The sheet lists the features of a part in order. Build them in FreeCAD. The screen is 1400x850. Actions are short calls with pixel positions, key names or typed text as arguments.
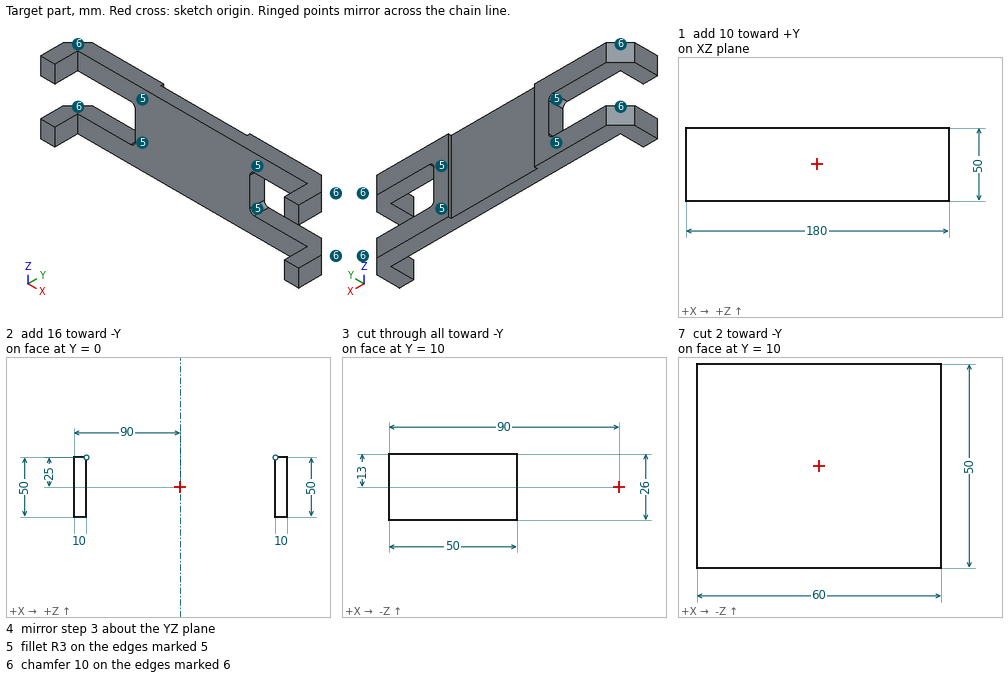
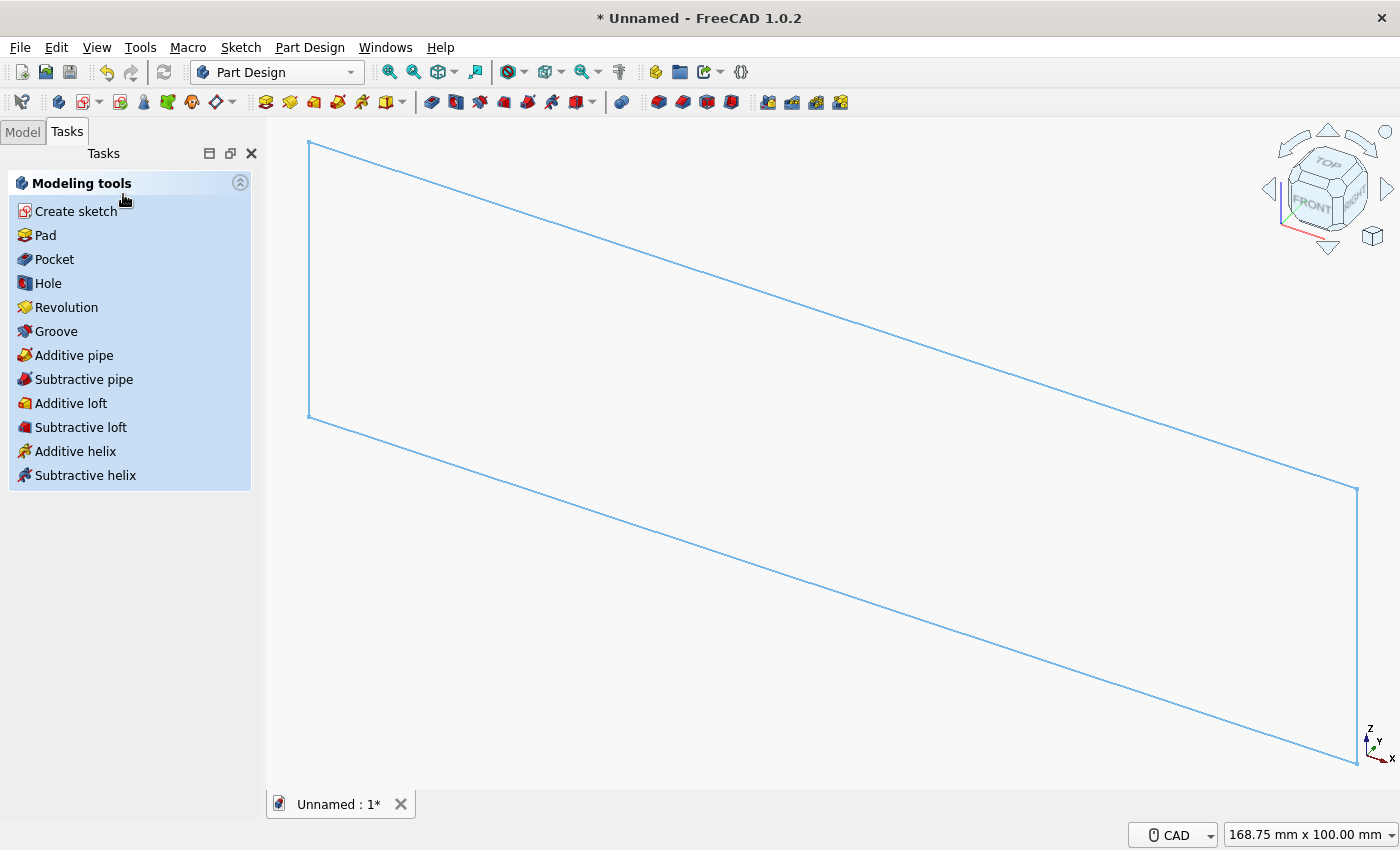
click(266, 102)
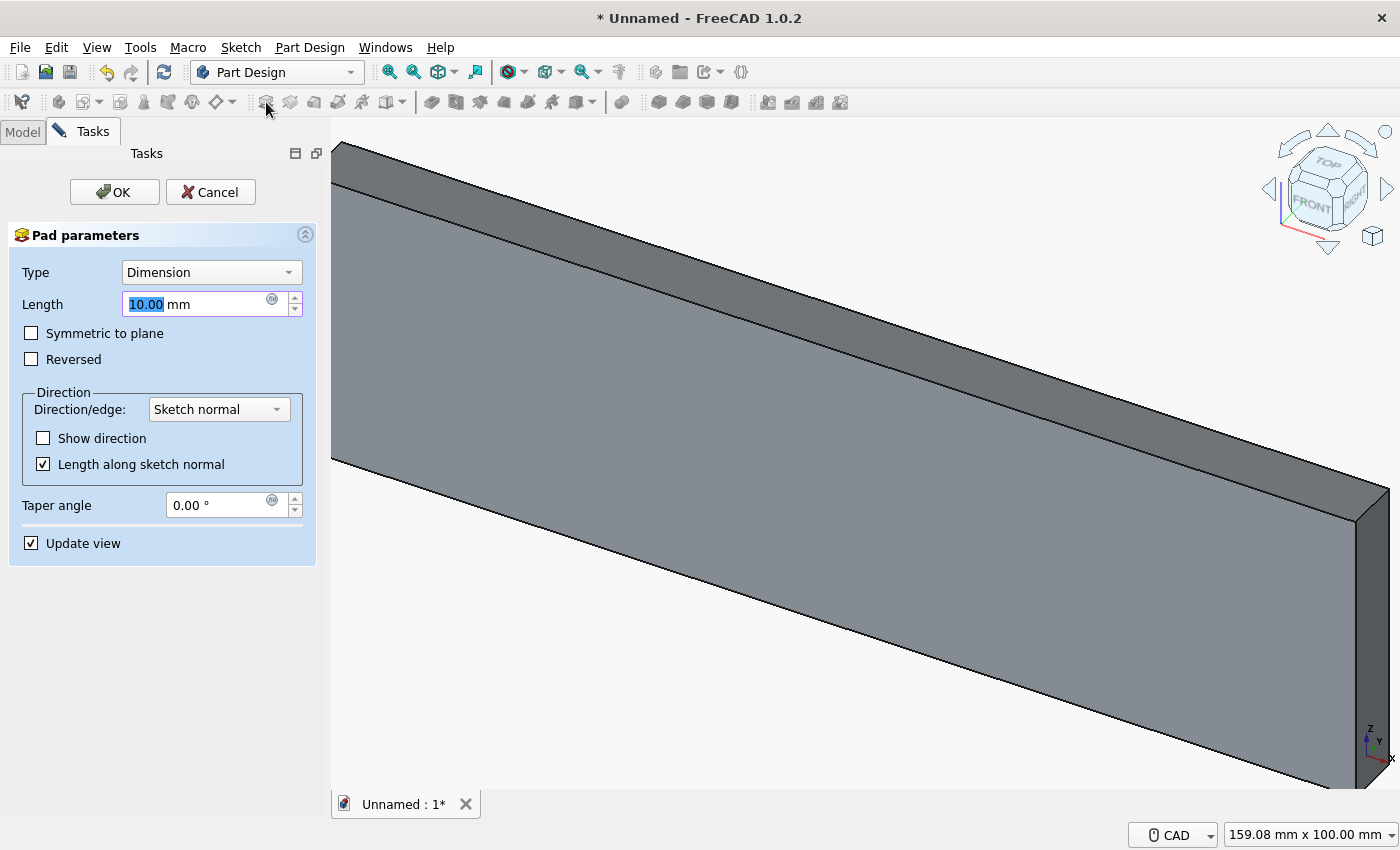
text(10)
key(Tab)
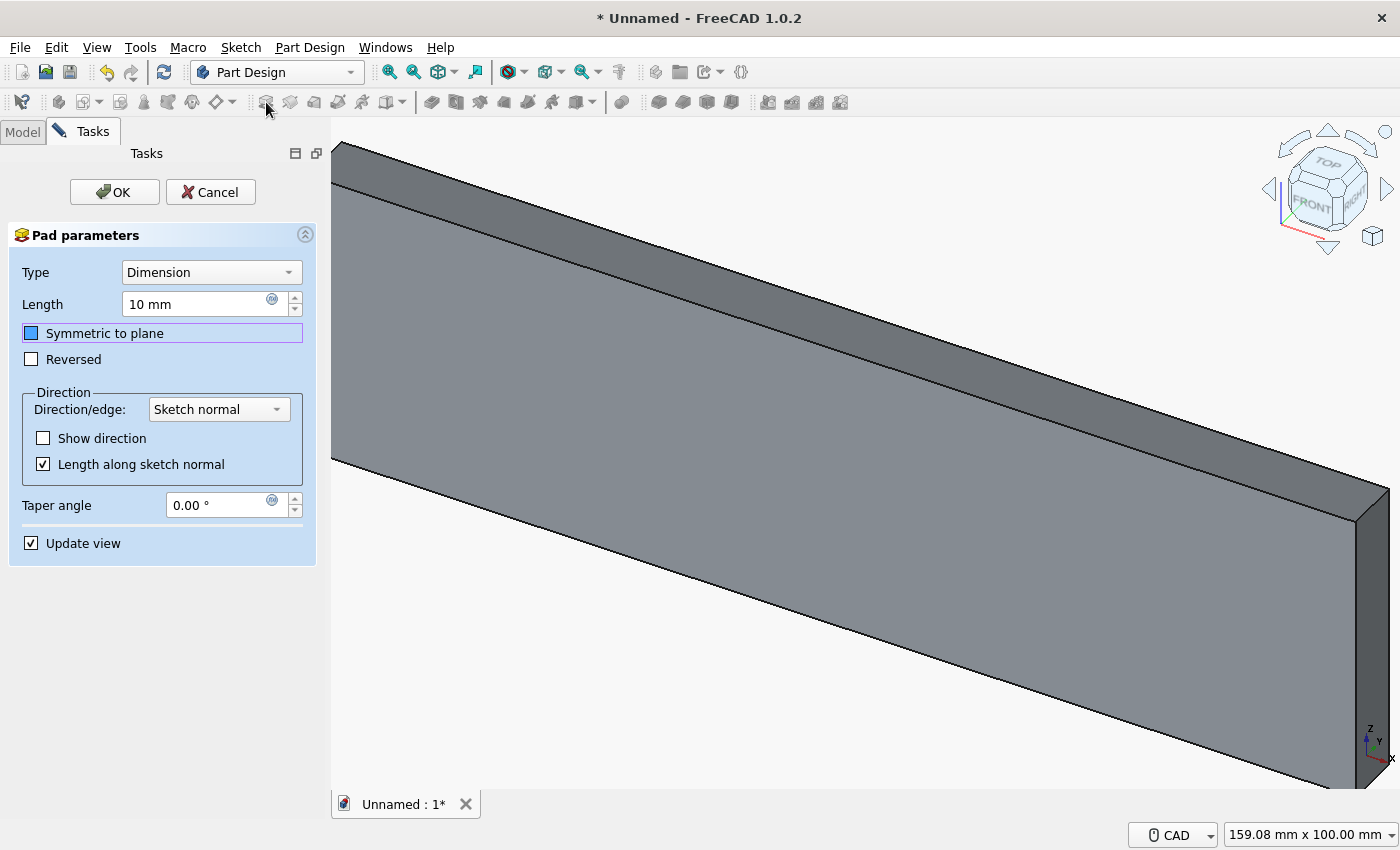
click(30, 359)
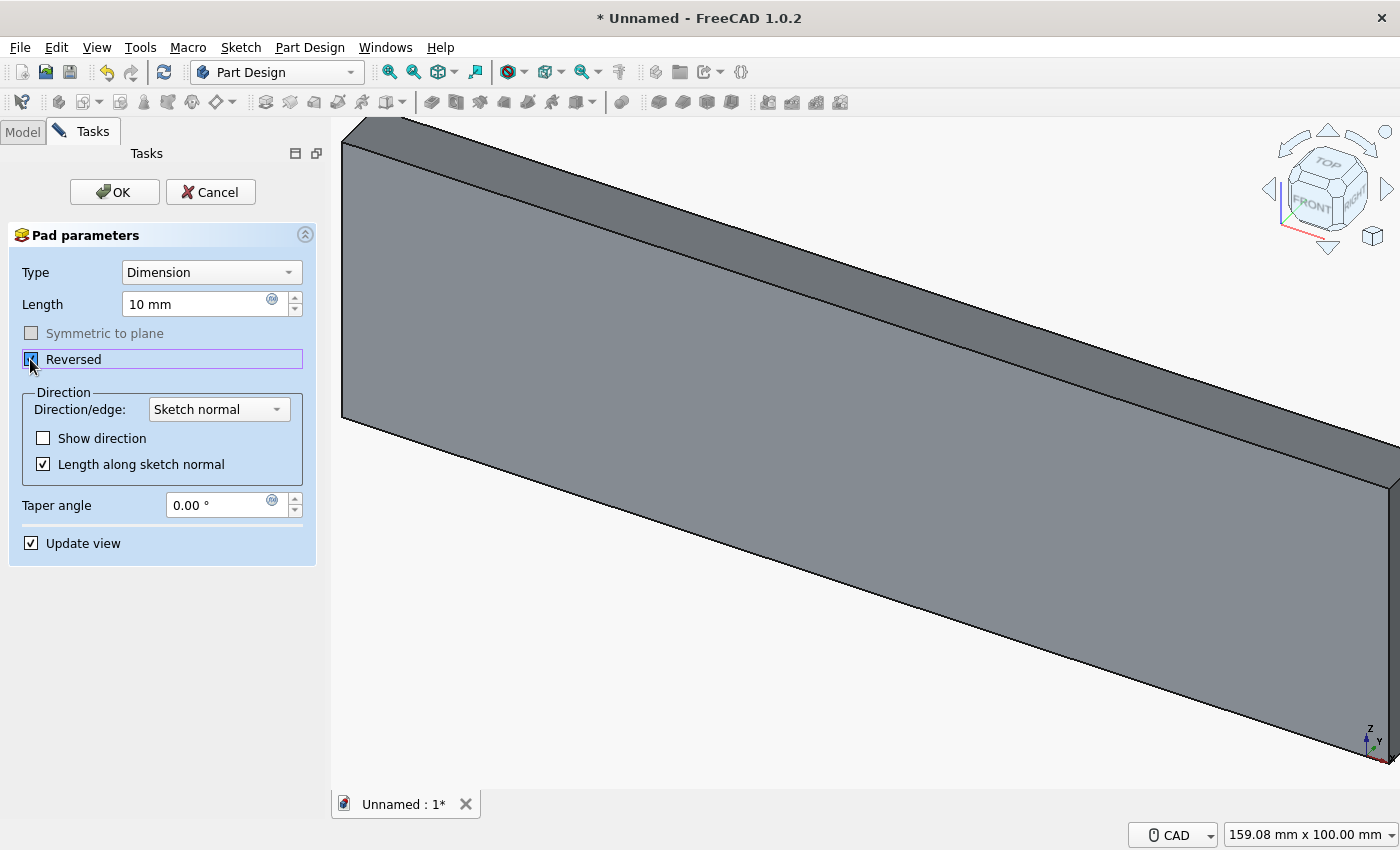
click(115, 192)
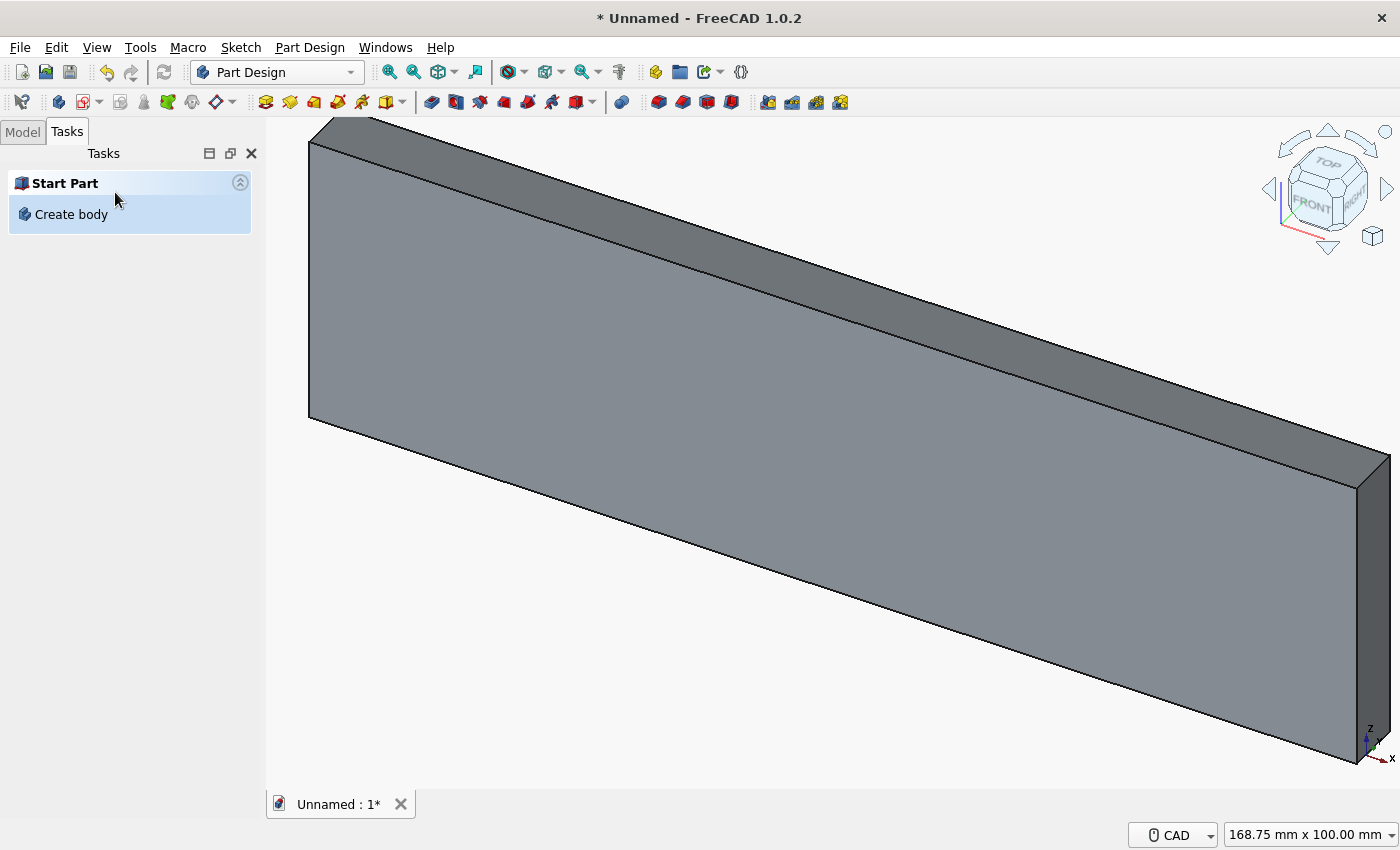
key(v)
key(f)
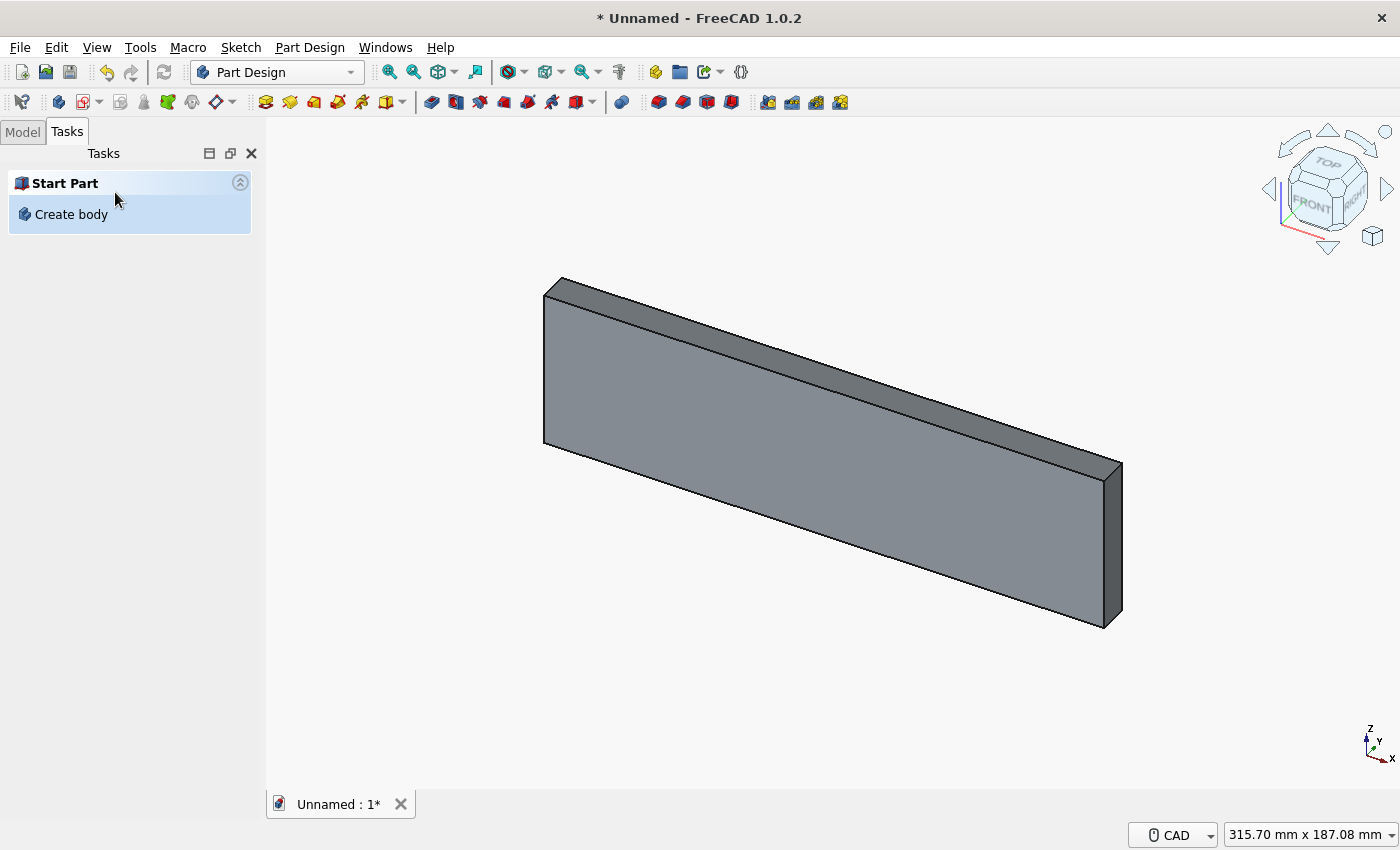
click(984, 514)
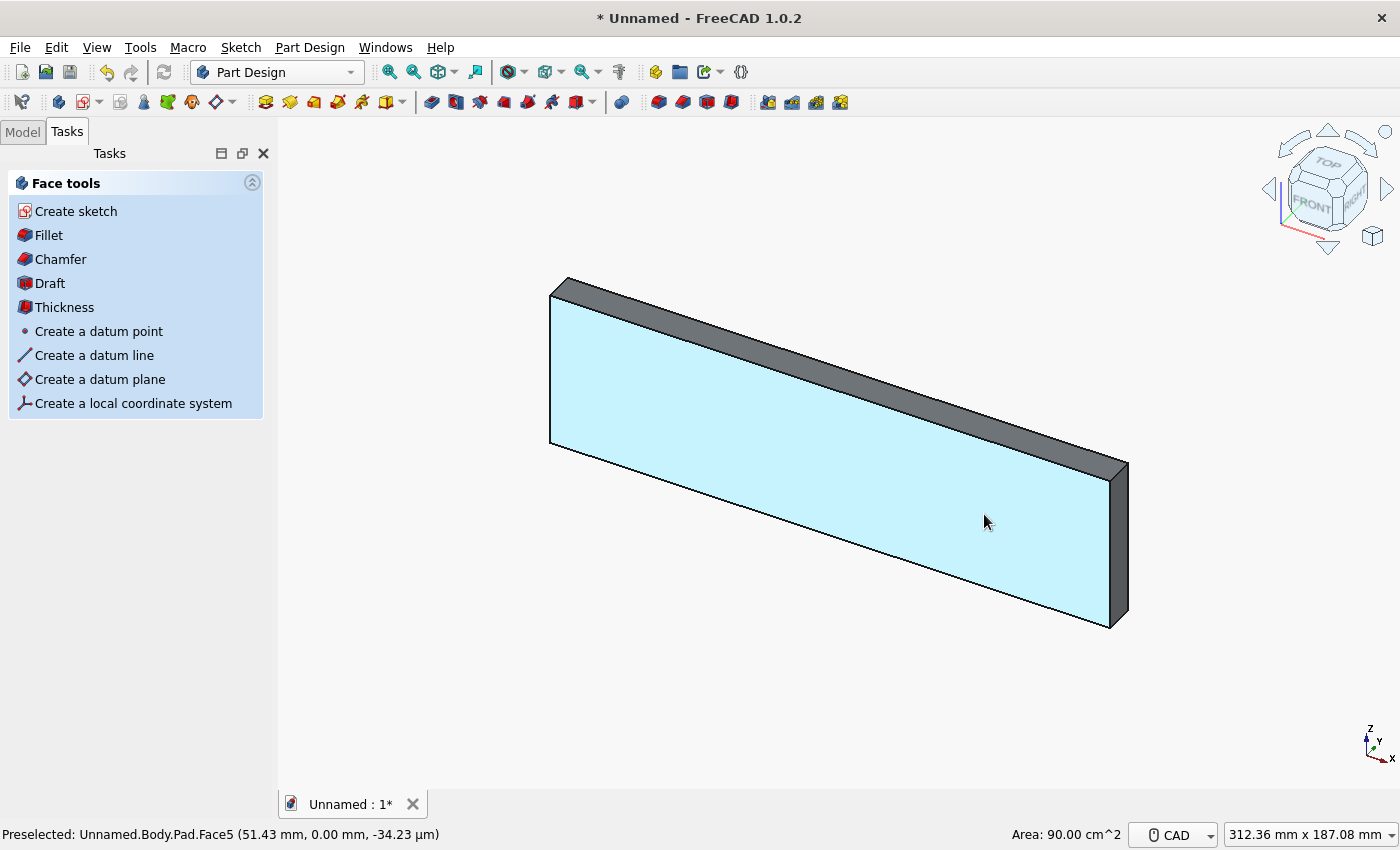
click(84, 102)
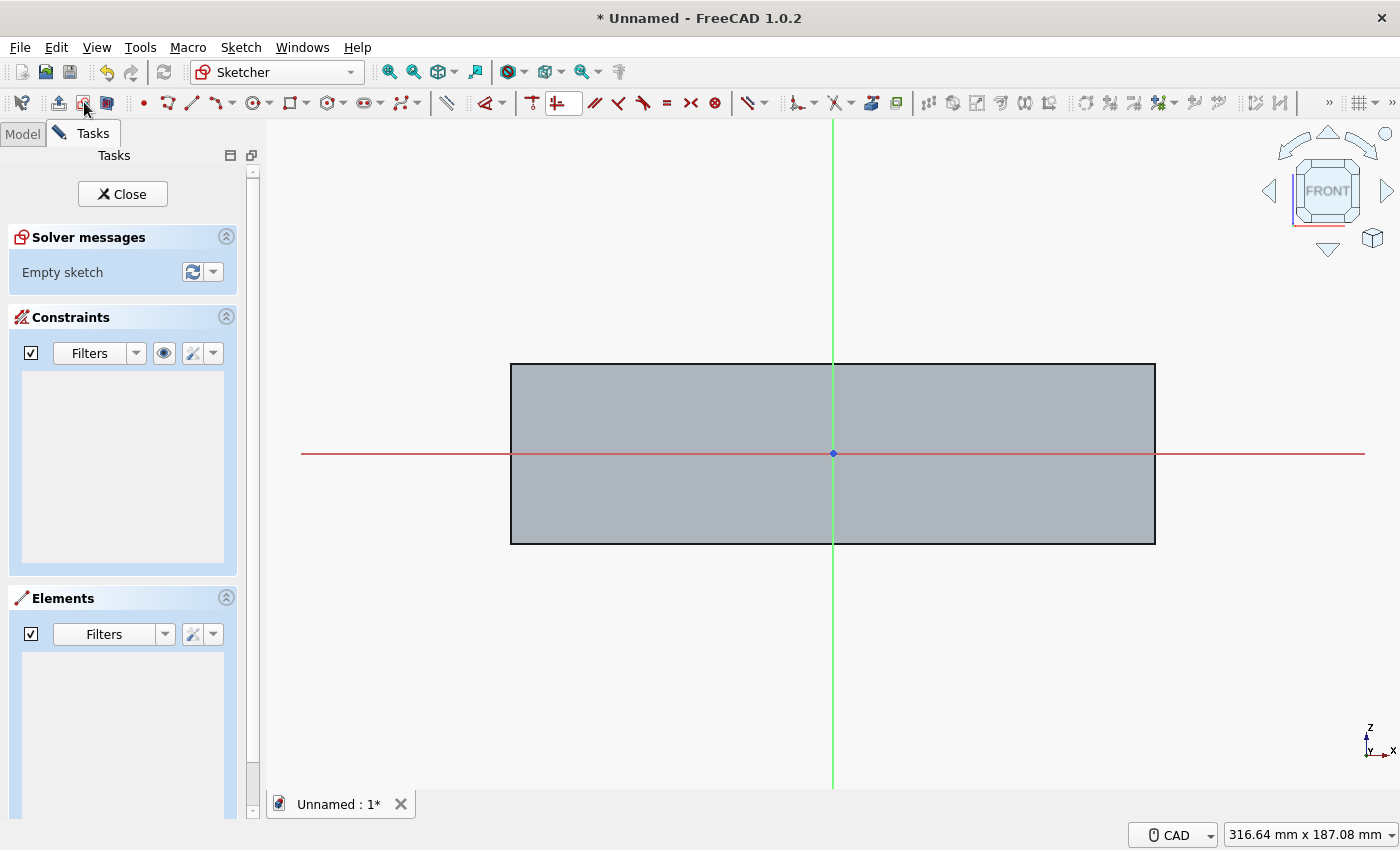
click(290, 104)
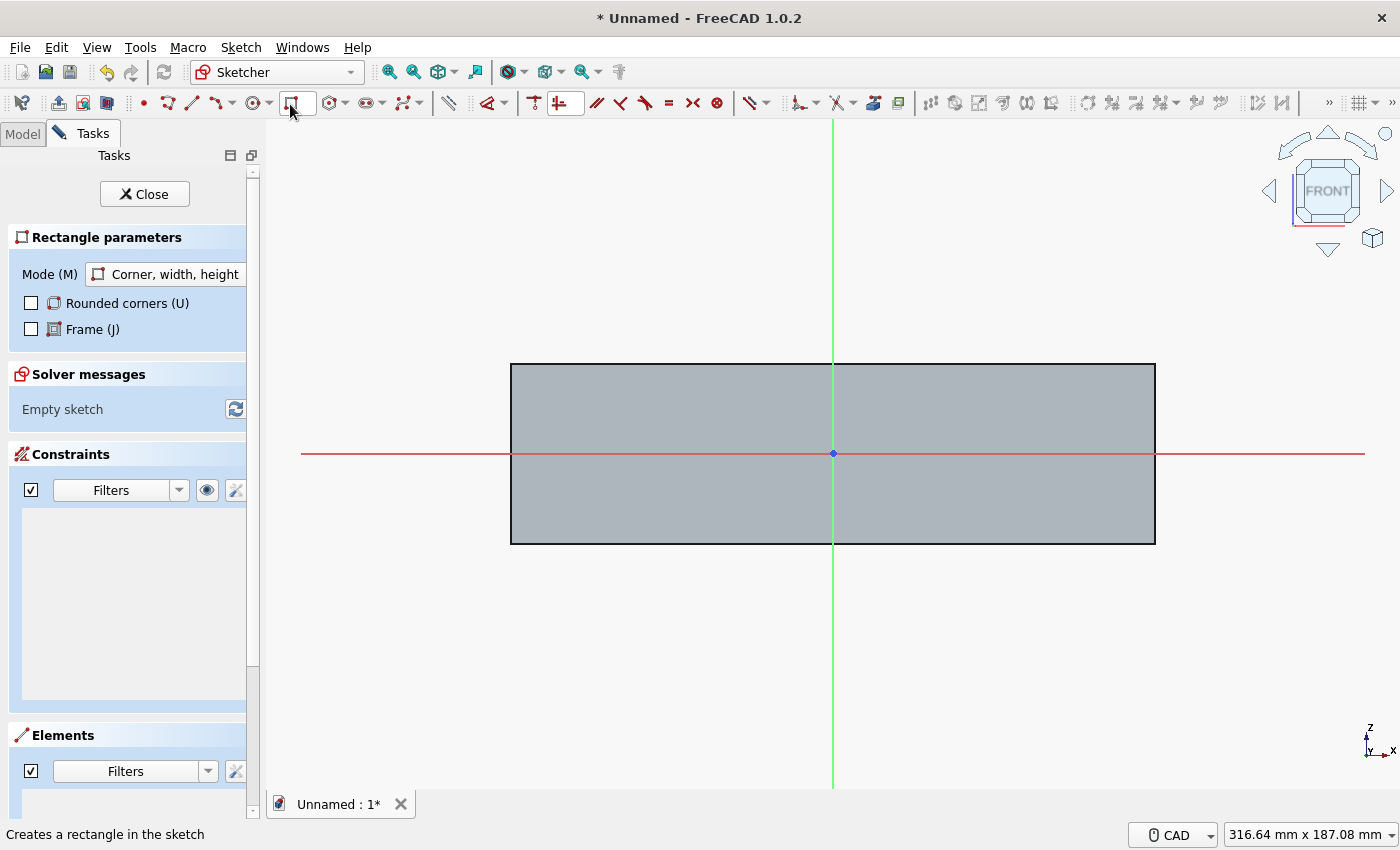
click(511, 364)
move(546, 544)